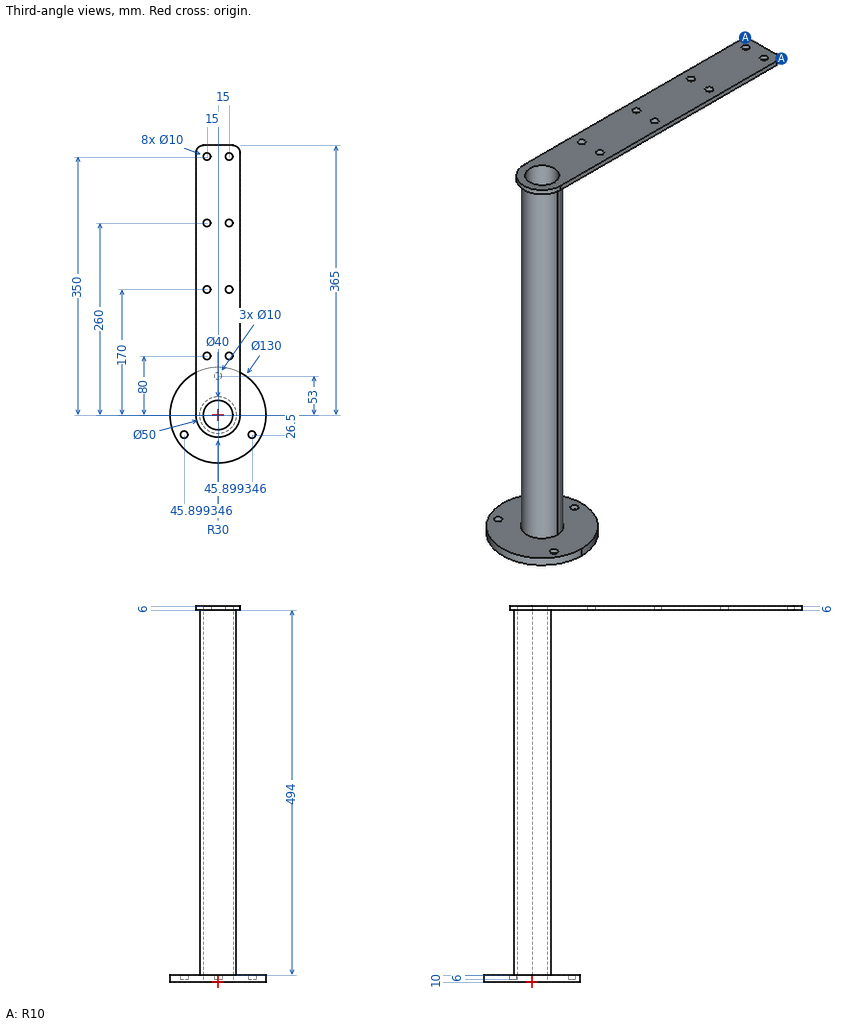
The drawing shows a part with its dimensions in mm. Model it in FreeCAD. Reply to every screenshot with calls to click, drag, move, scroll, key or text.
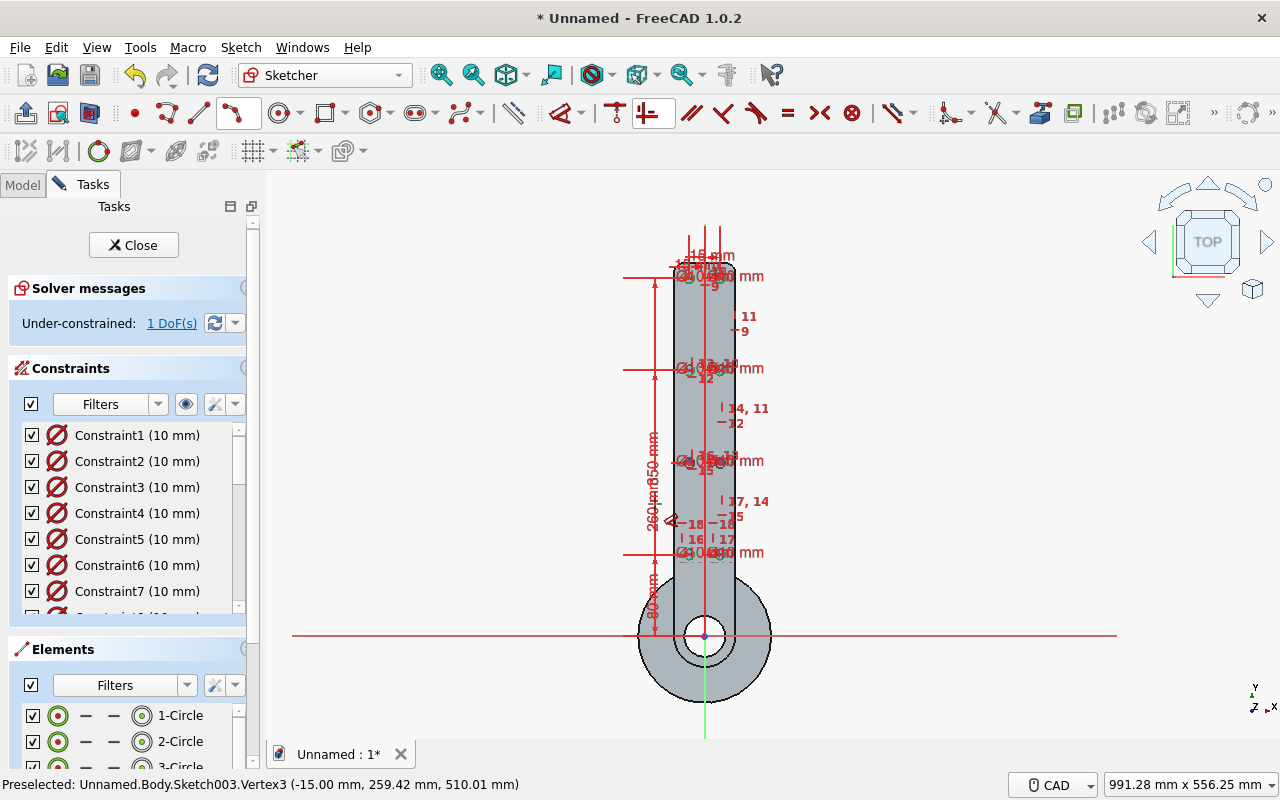
click(689, 463)
click(655, 550)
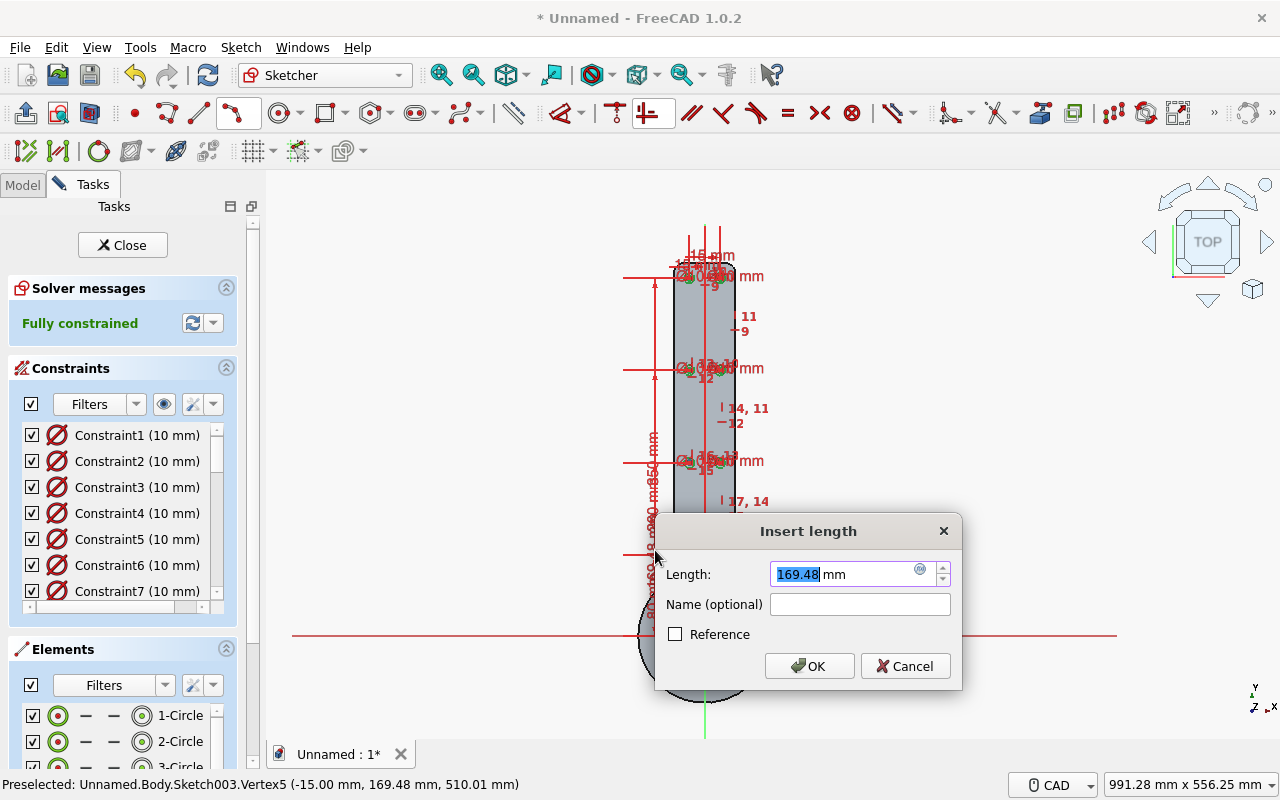
text(170)
key(Return)
key(Escape)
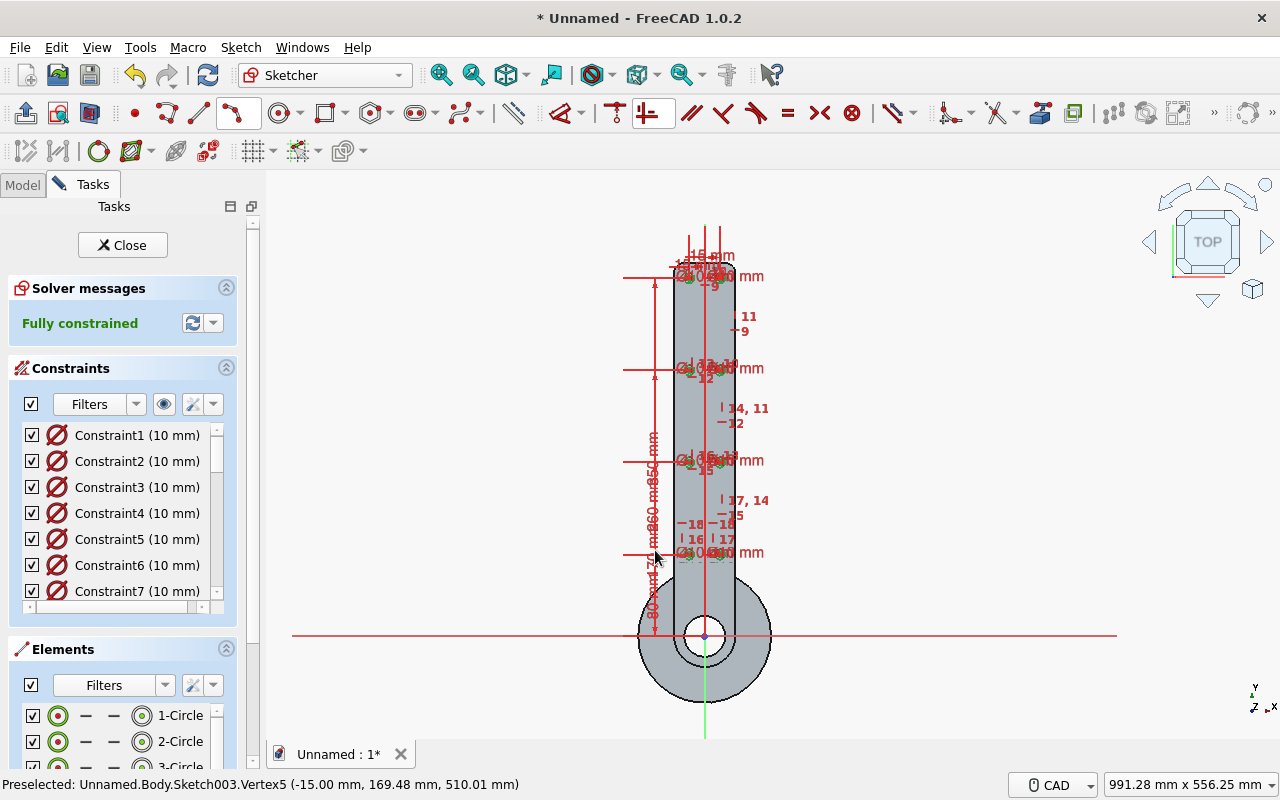
click(123, 245)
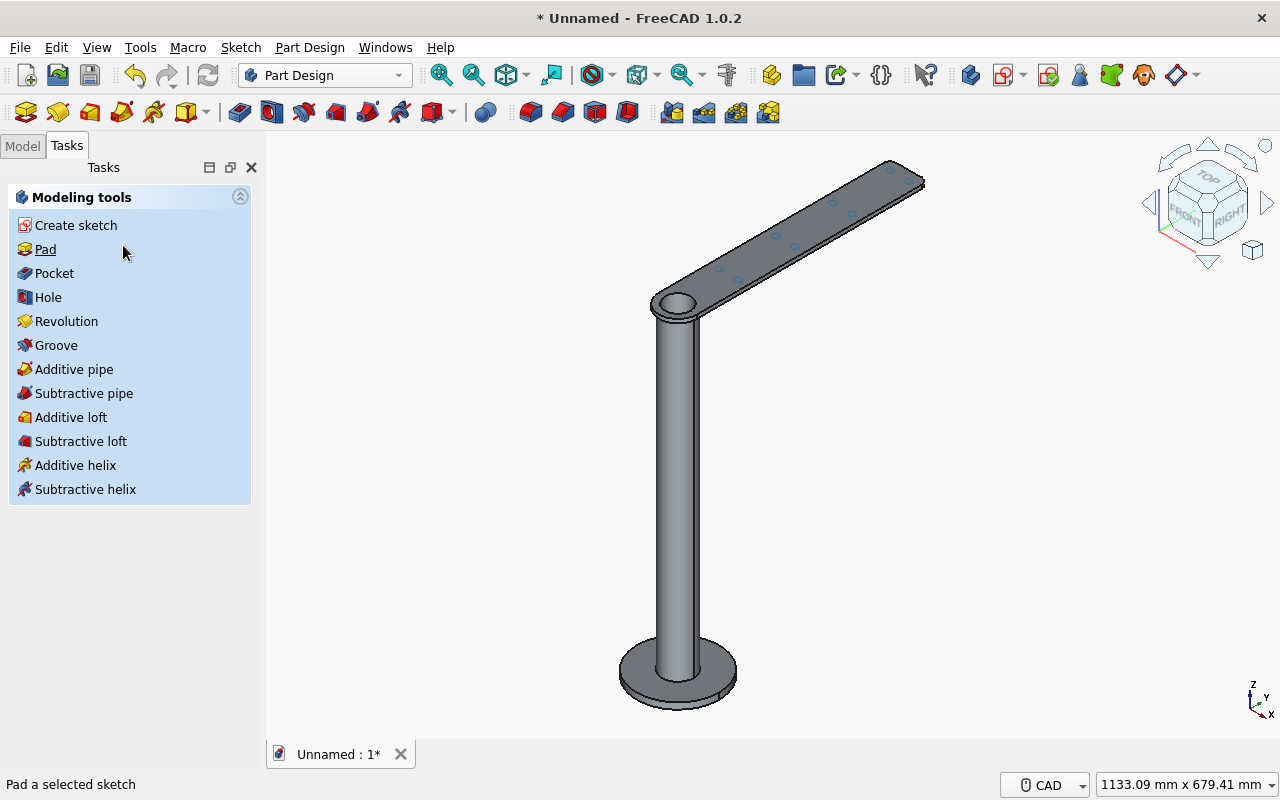
click(240, 112)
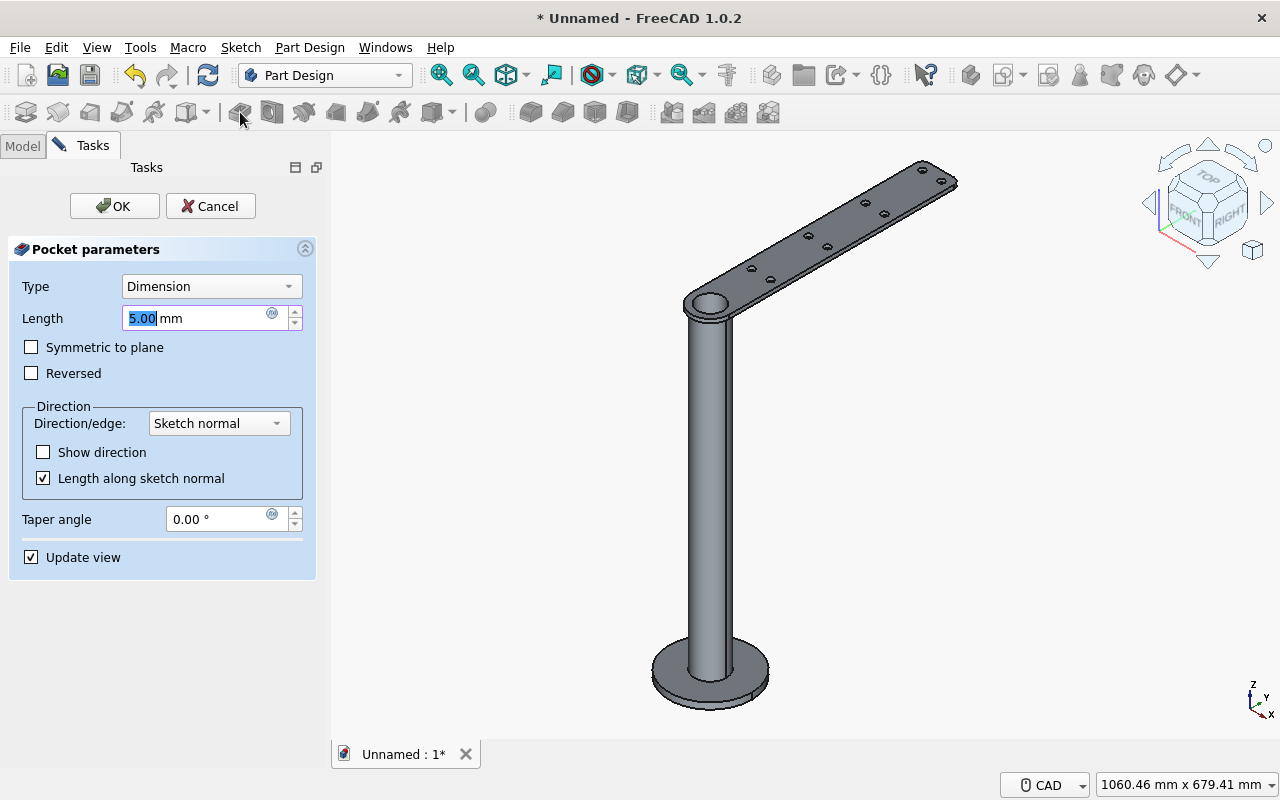
text(6)
key(Tab)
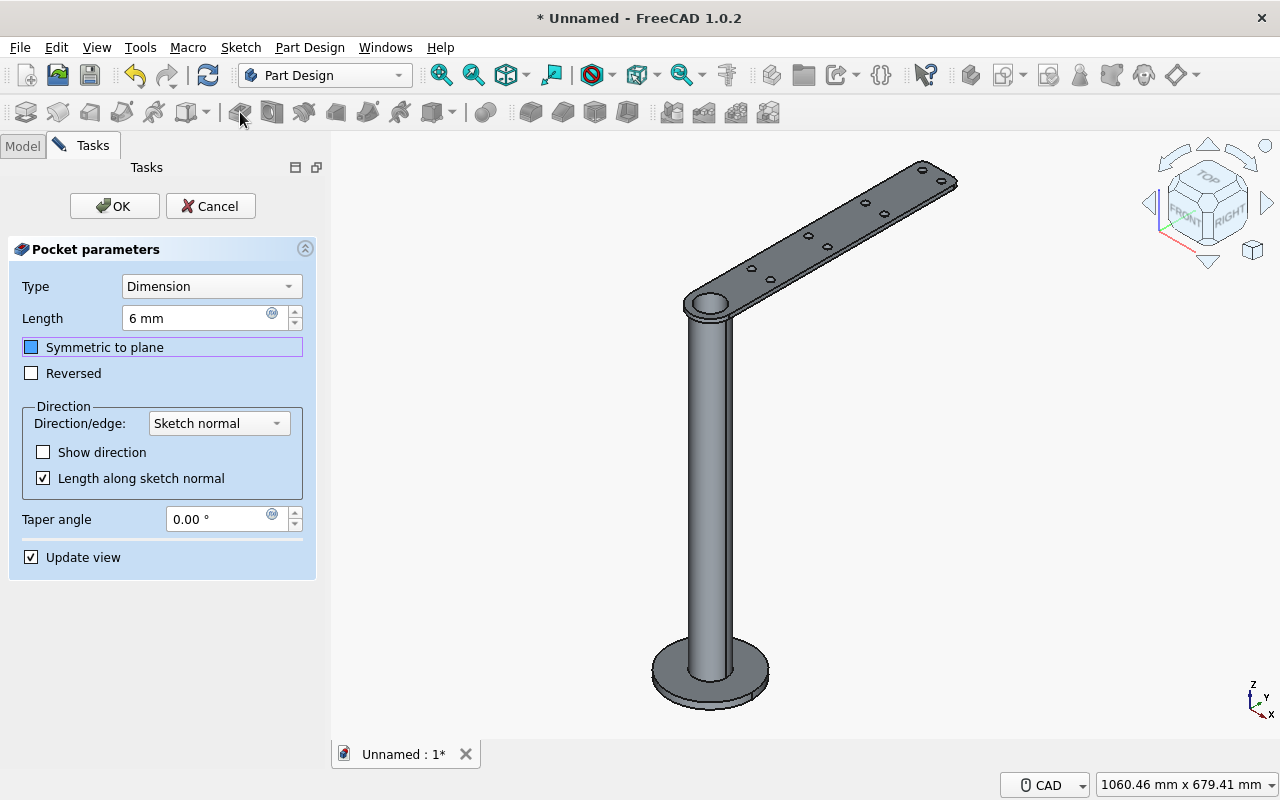
click(115, 206)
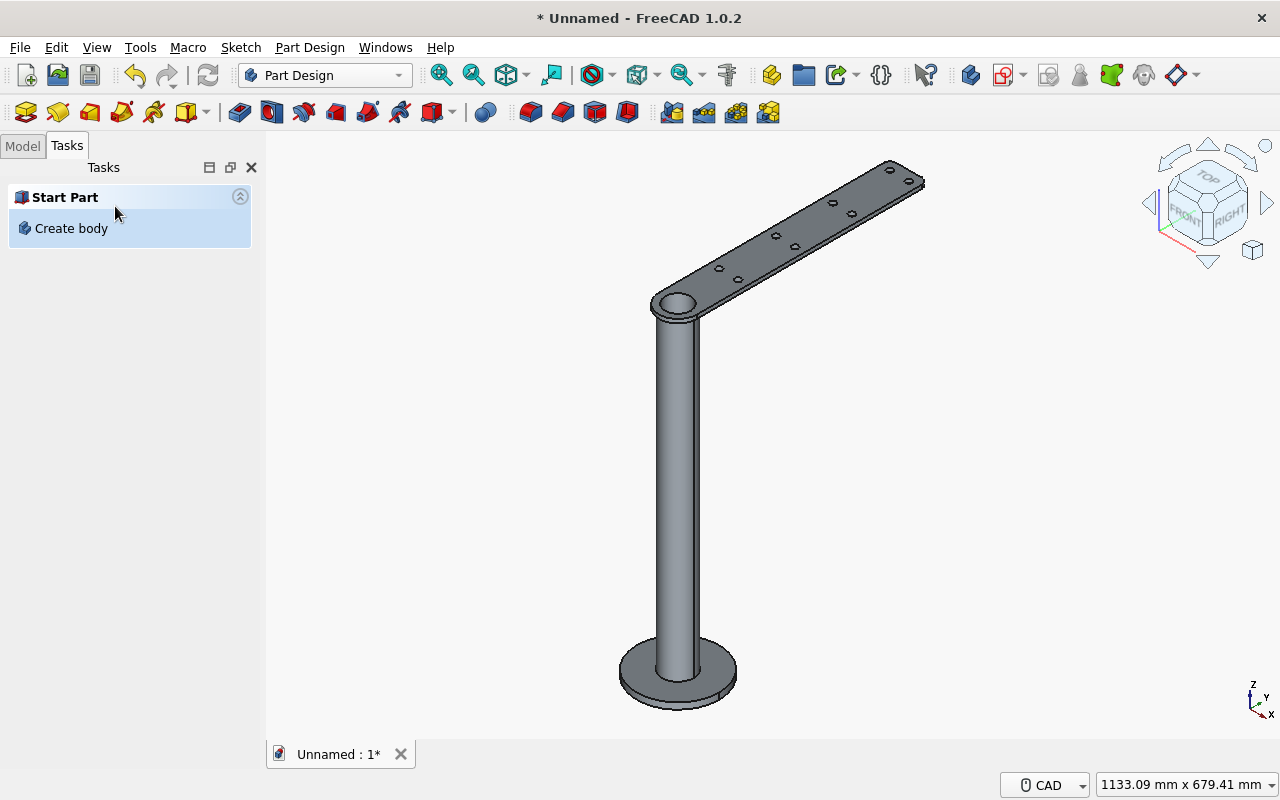
click(713, 675)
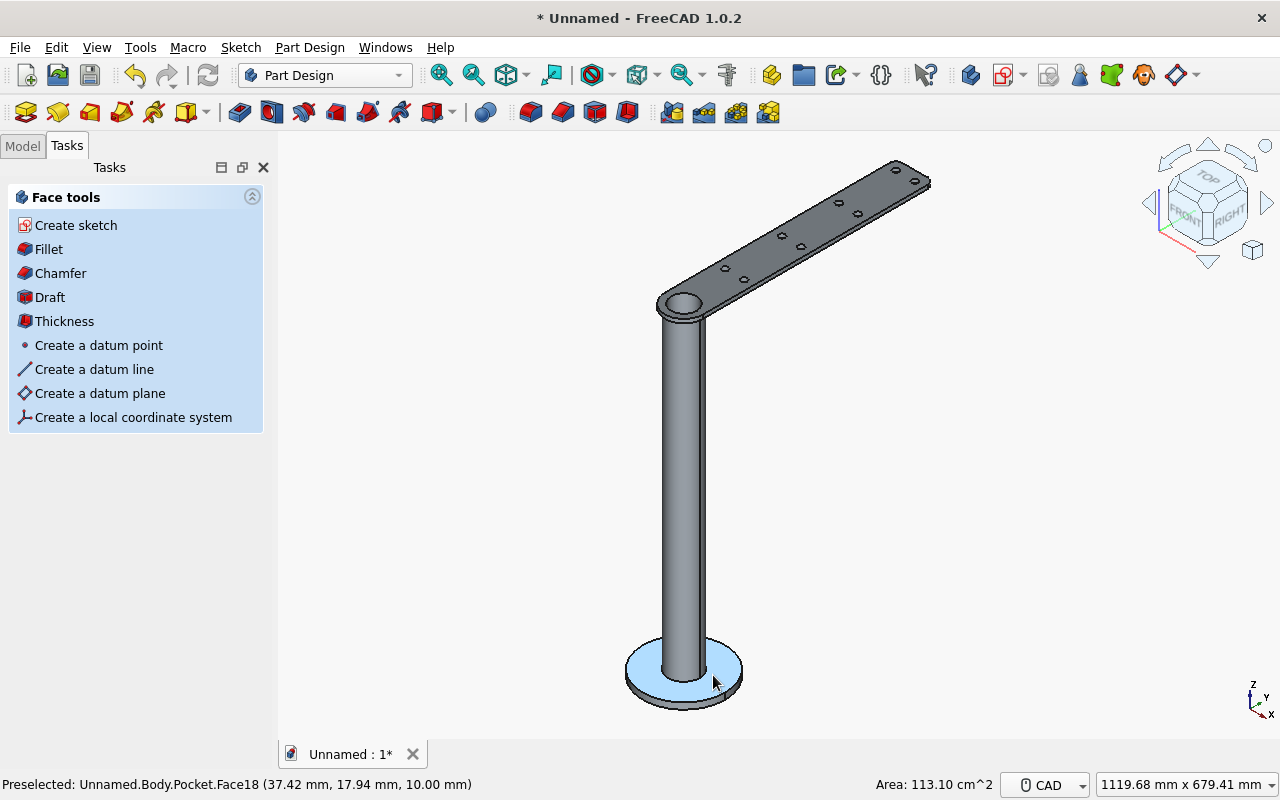
click(1004, 76)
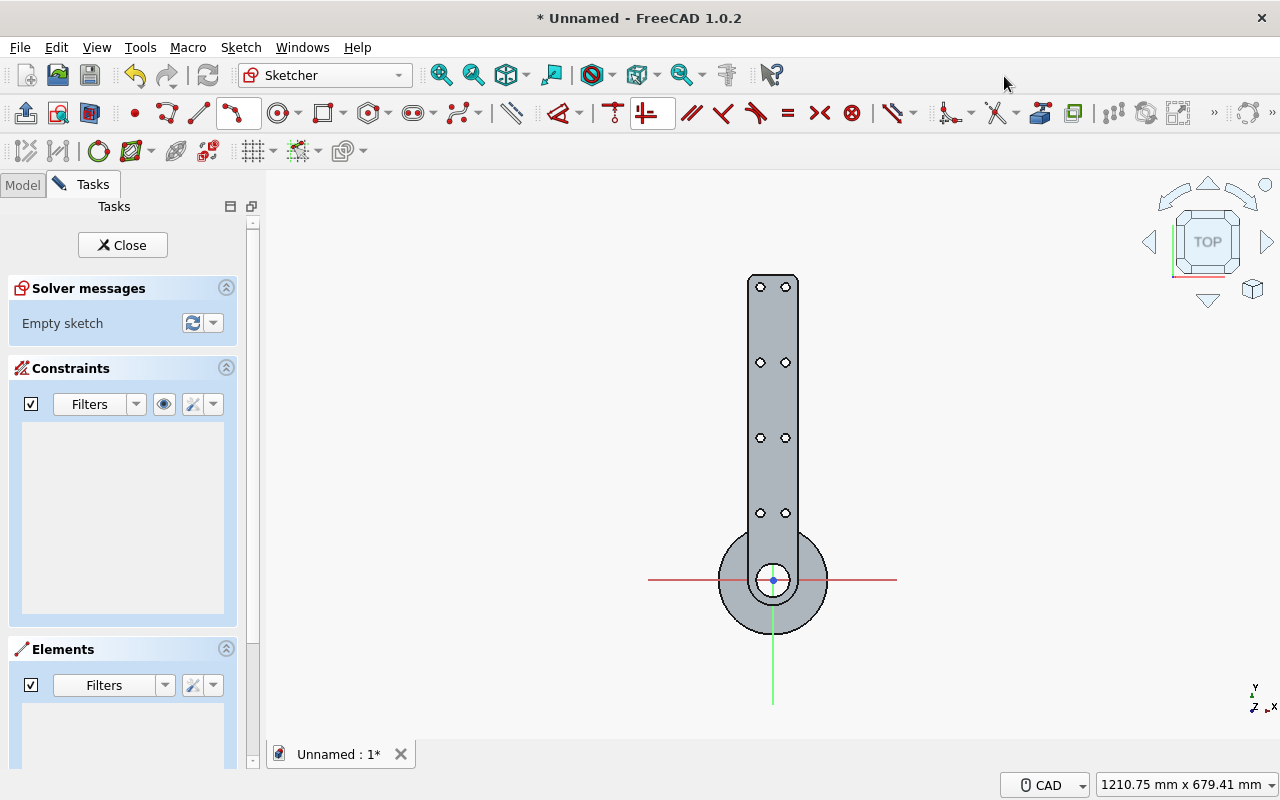
scroll(790, 598, up, 8)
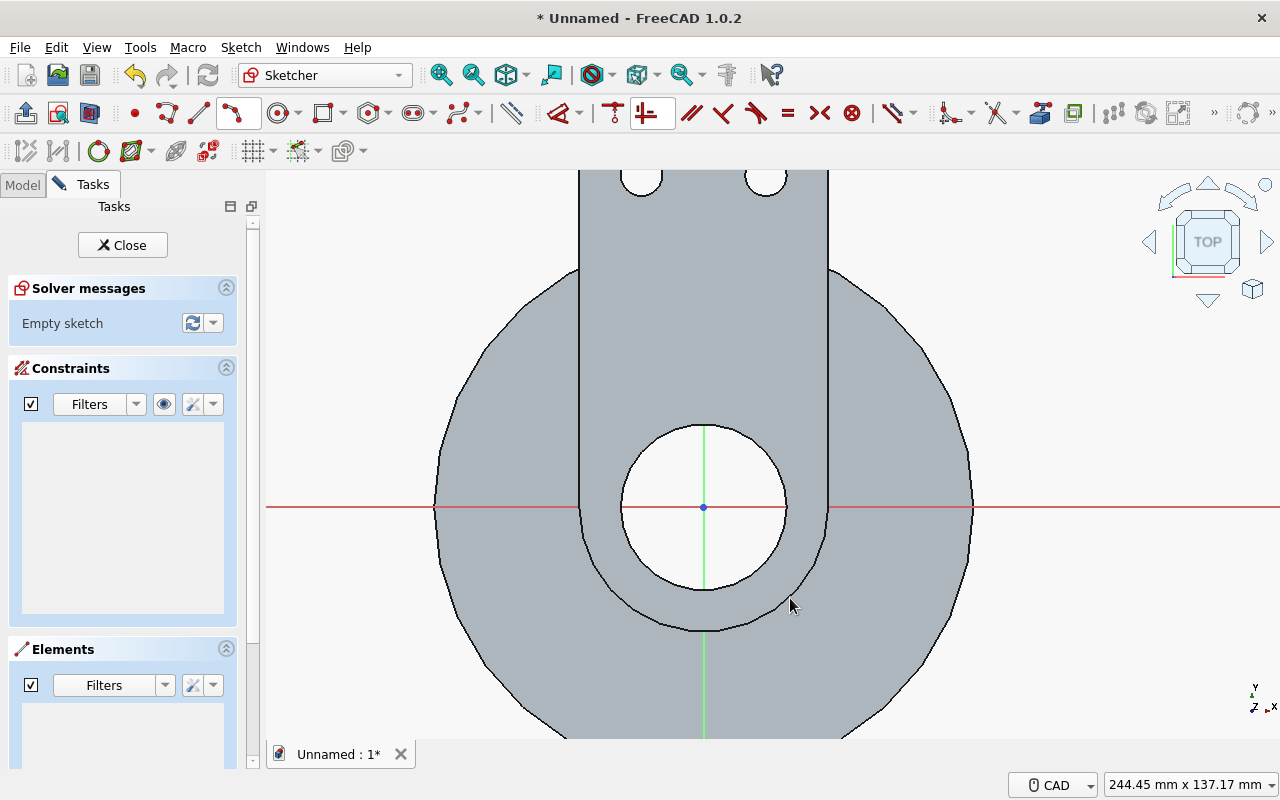
click(278, 114)